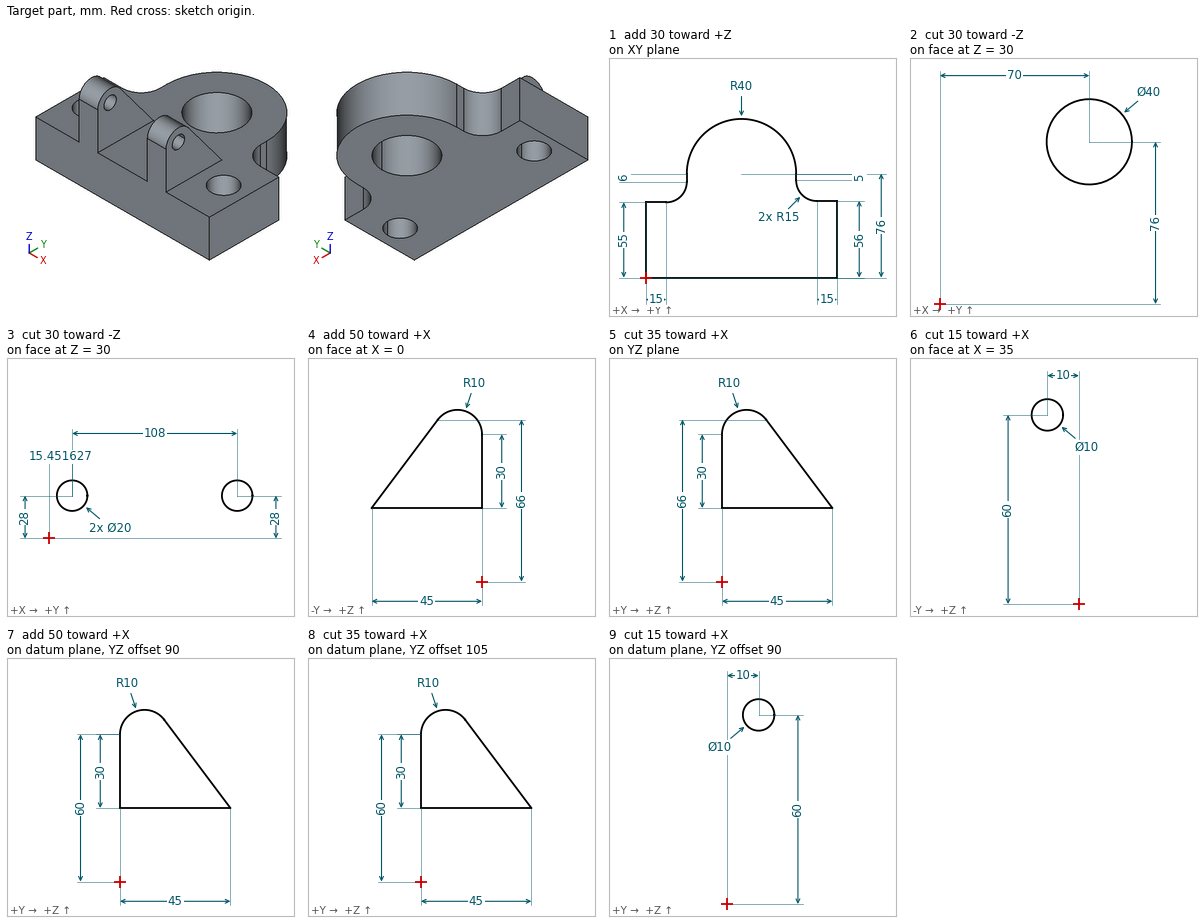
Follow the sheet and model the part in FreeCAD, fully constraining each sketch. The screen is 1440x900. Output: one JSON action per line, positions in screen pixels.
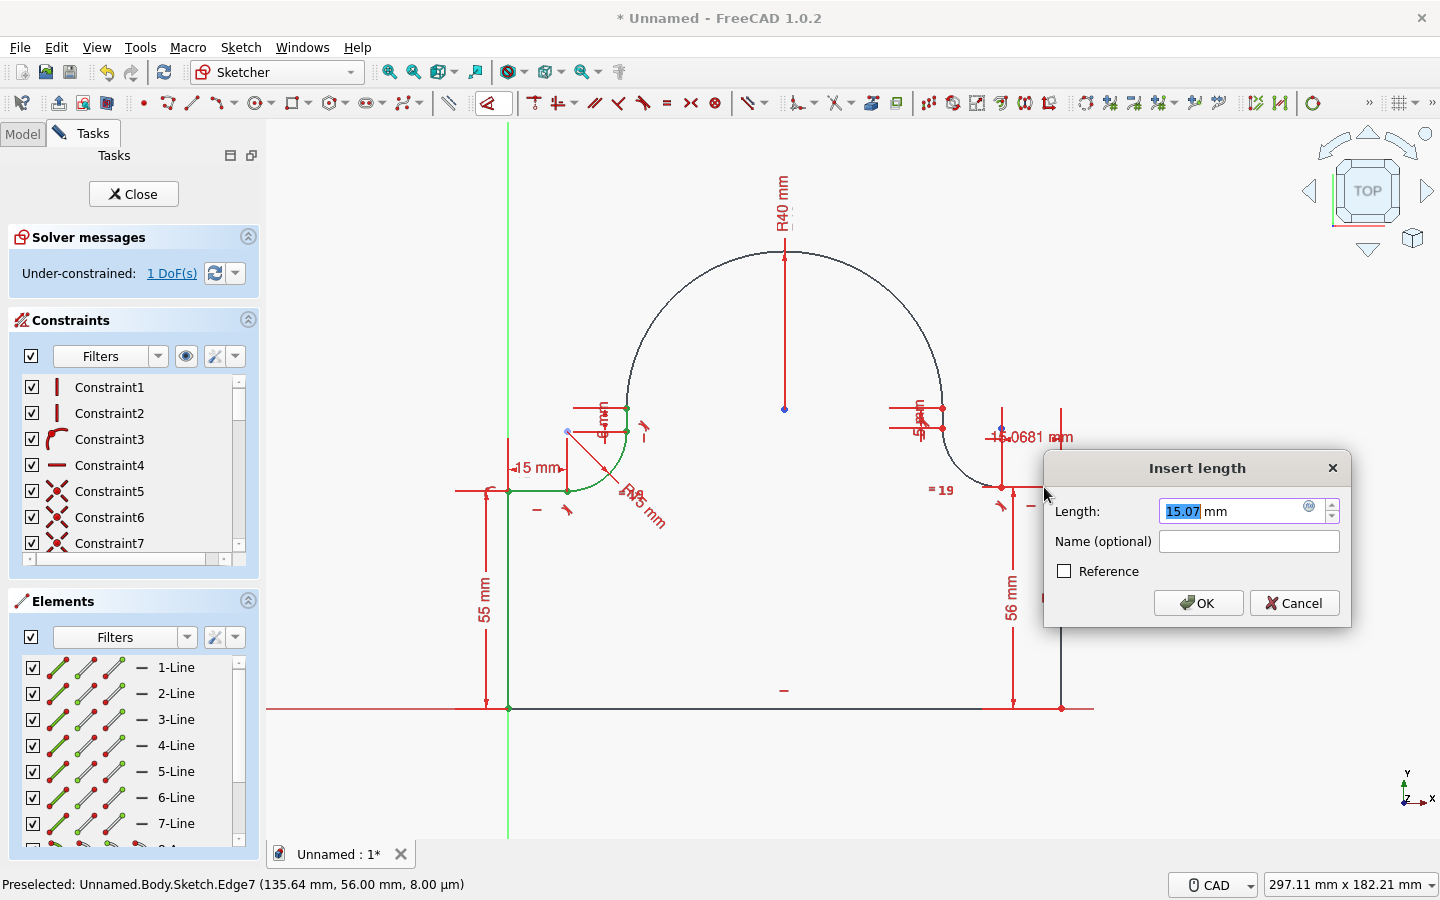
{"action": "type", "text": "15"}
{"action": "key", "text": "Return"}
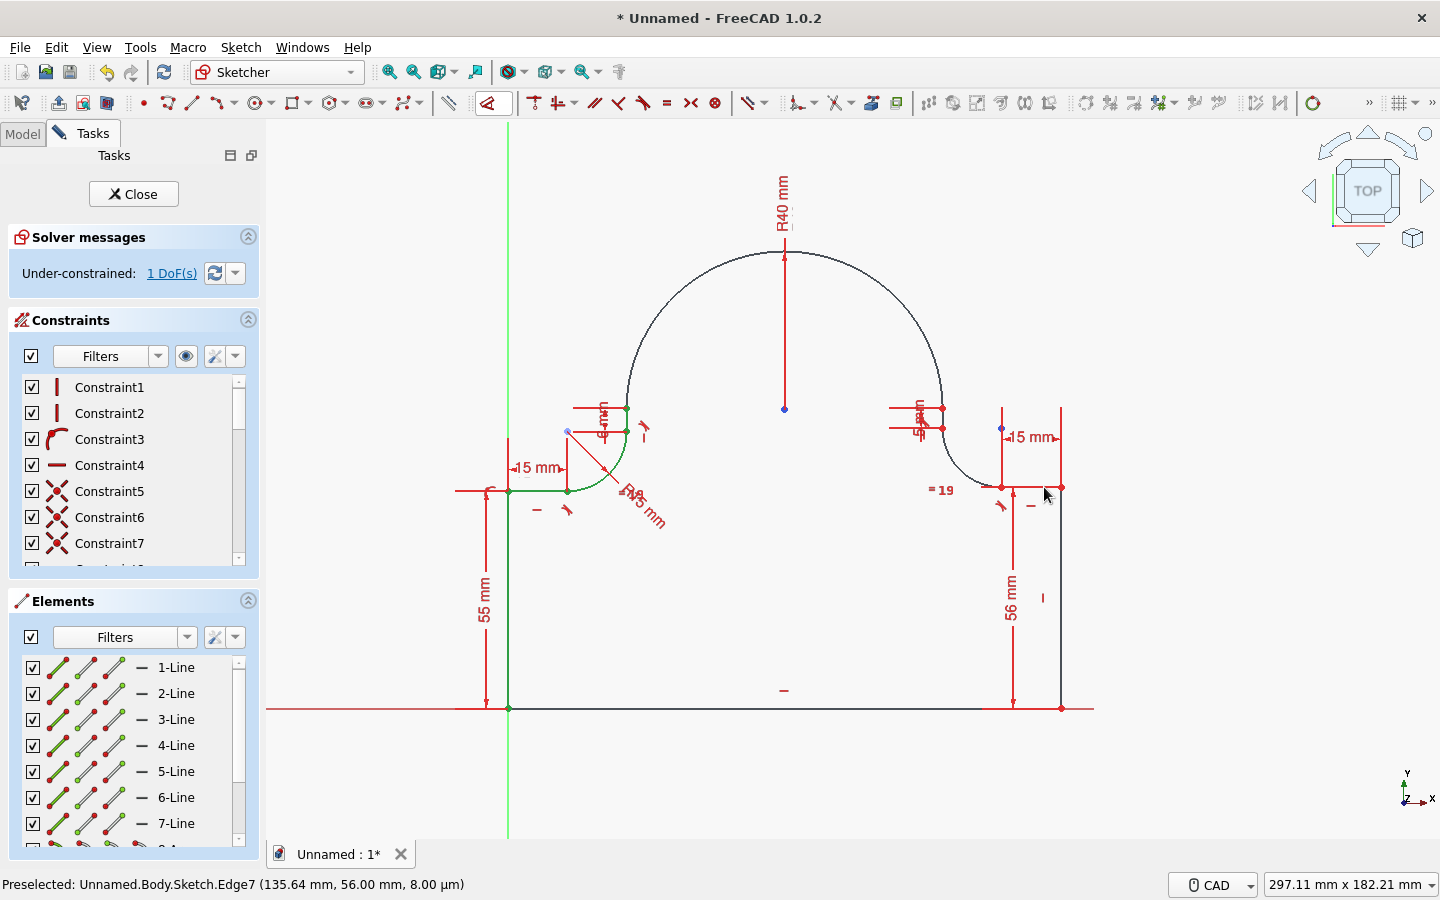
{"action": "left_click", "coordinate": [785, 410]}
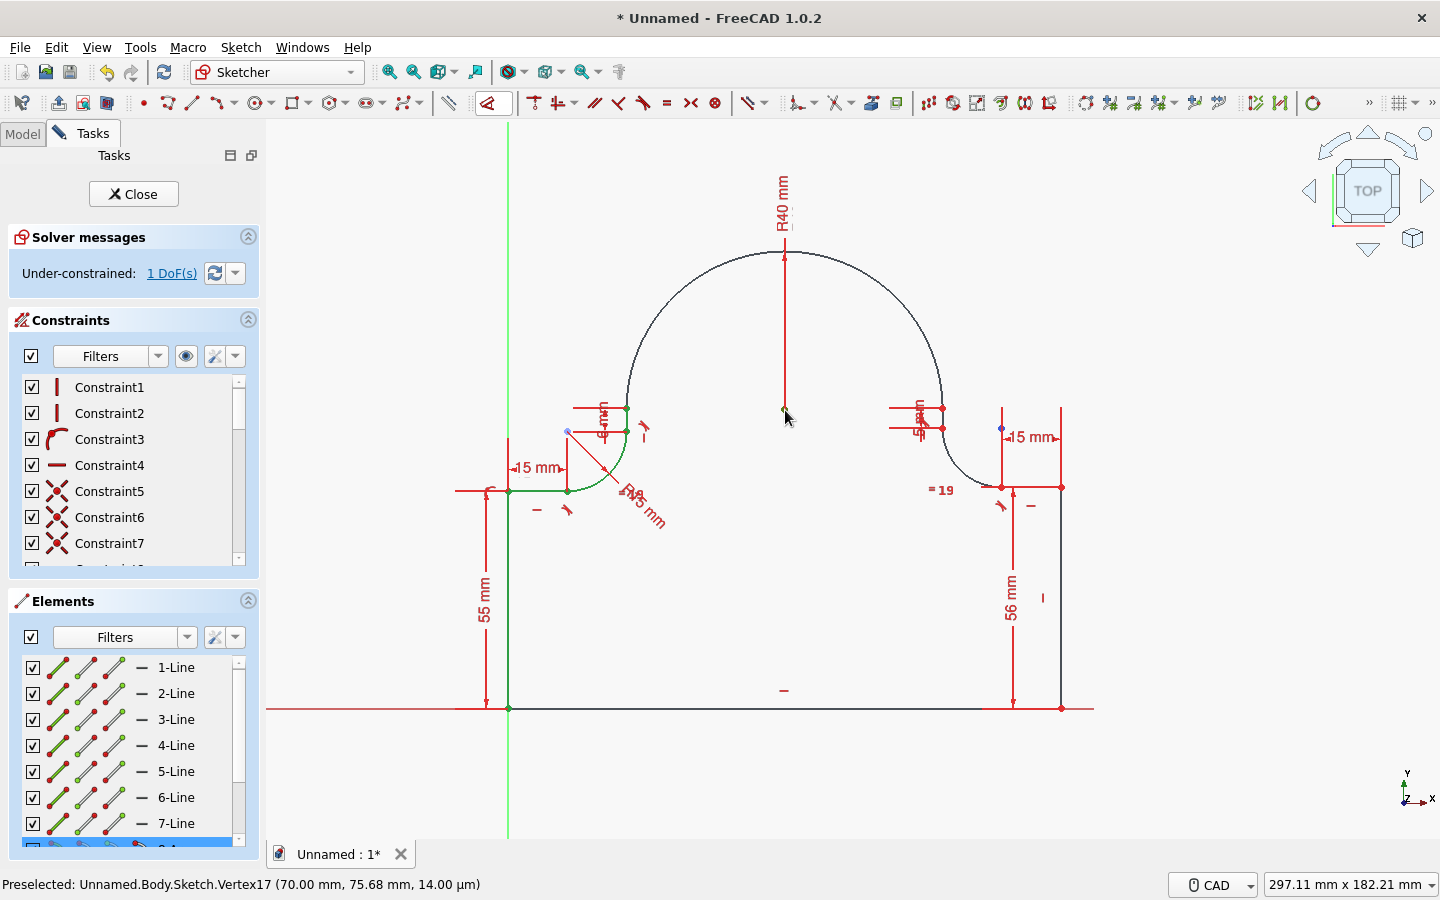
{"action": "key", "text": "i"}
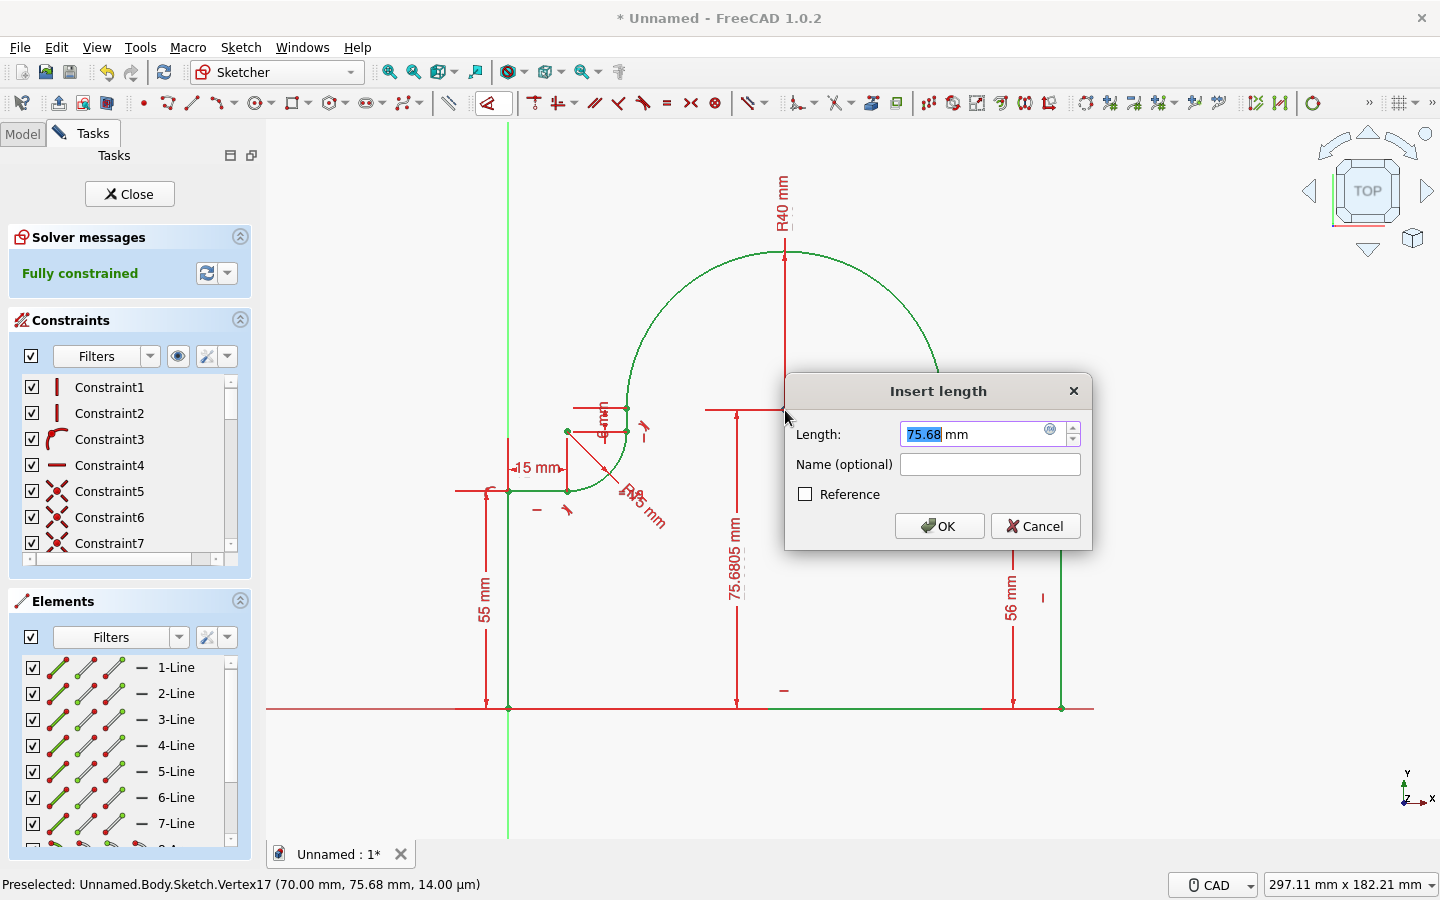
{"action": "type", "text": "76"}
{"action": "key", "text": "Return"}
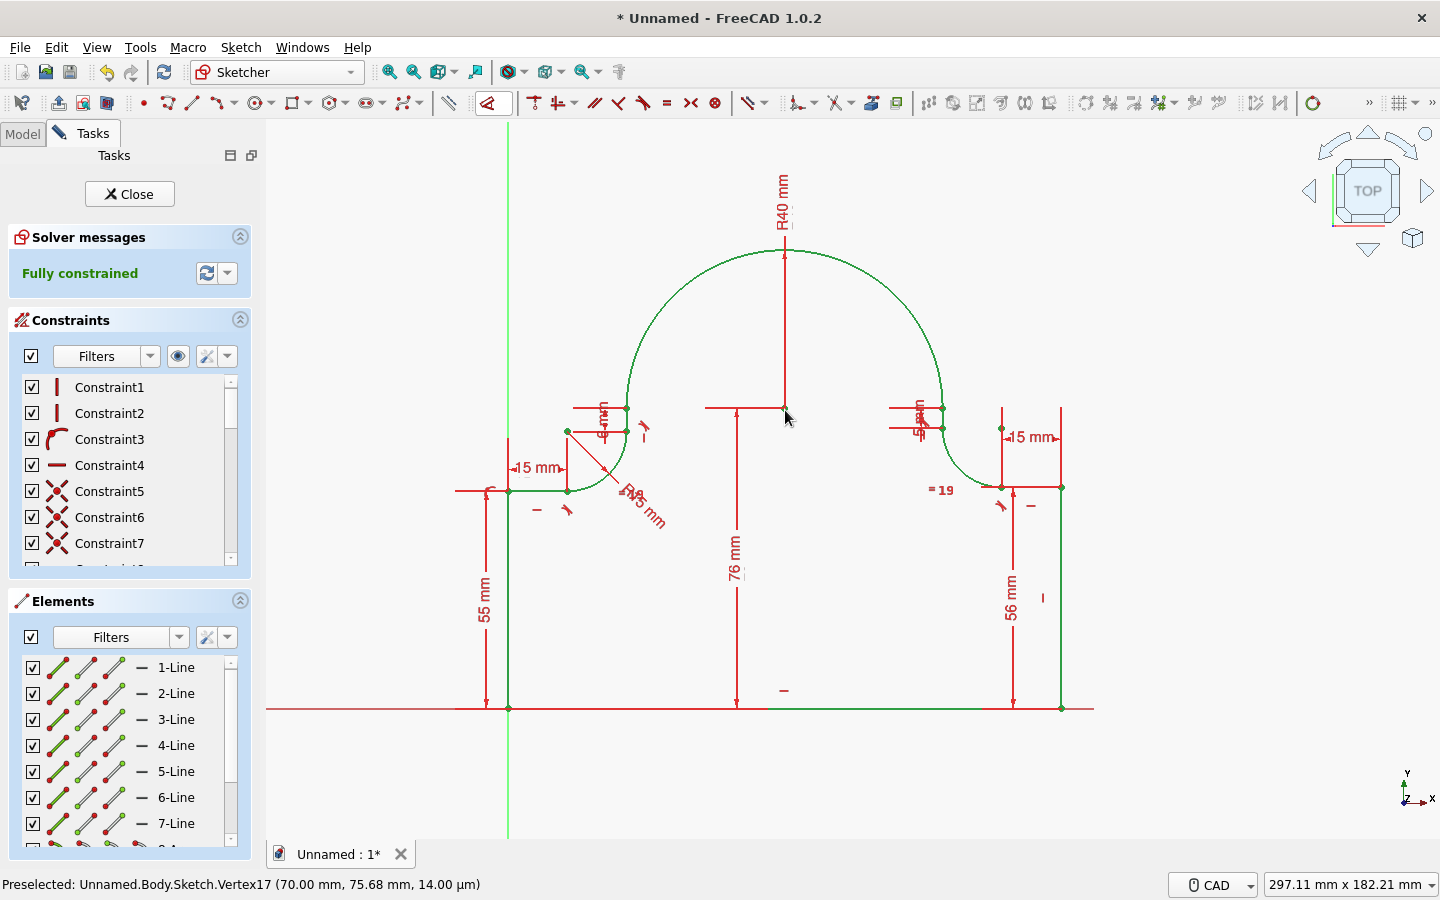
{"action": "left_click", "coordinate": [130, 194]}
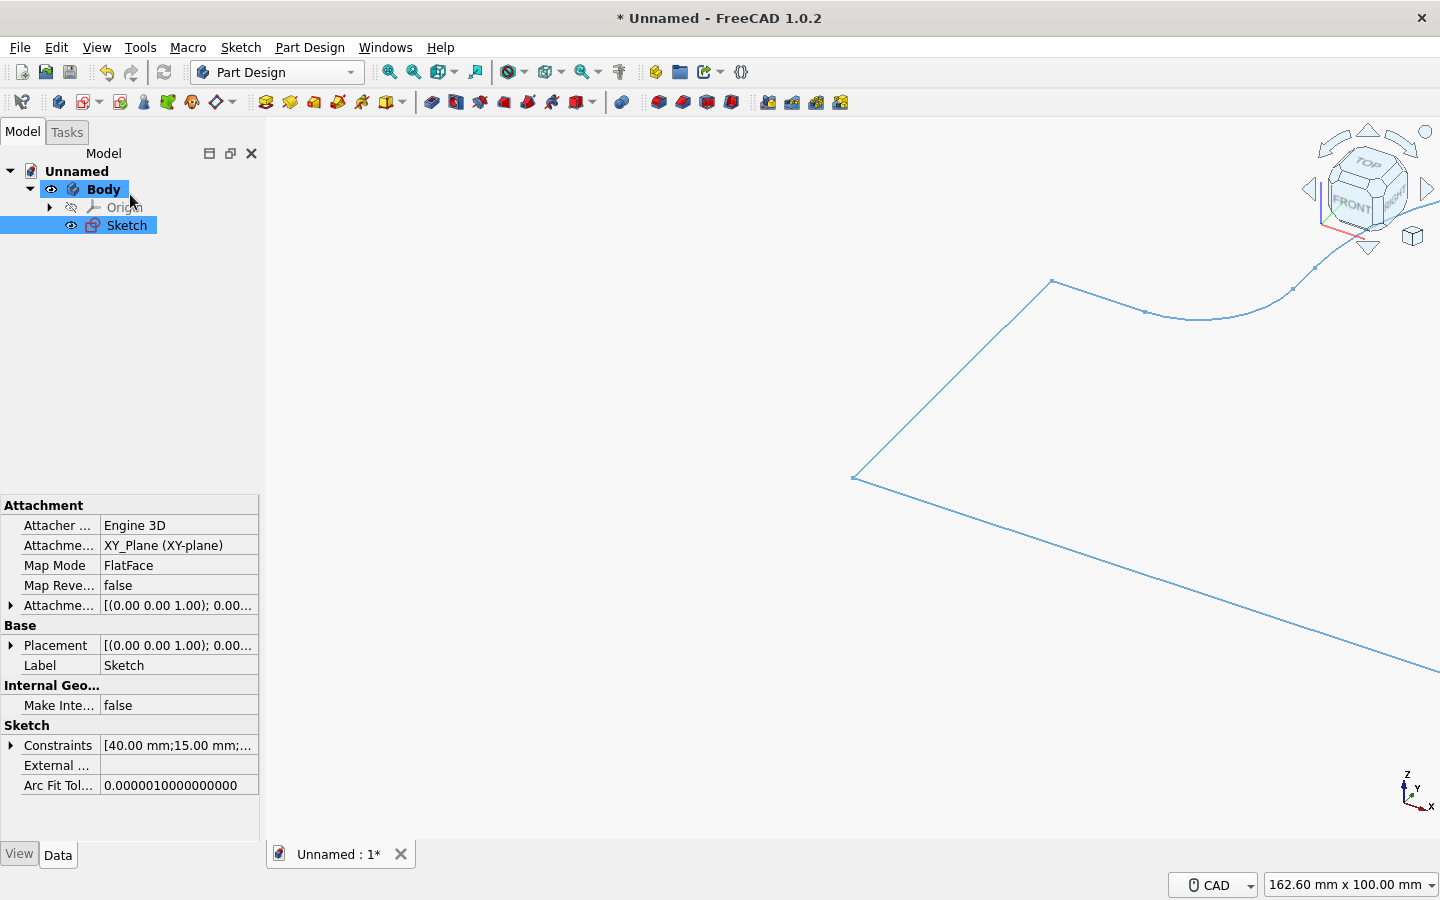
{"action": "left_click", "coordinate": [266, 102]}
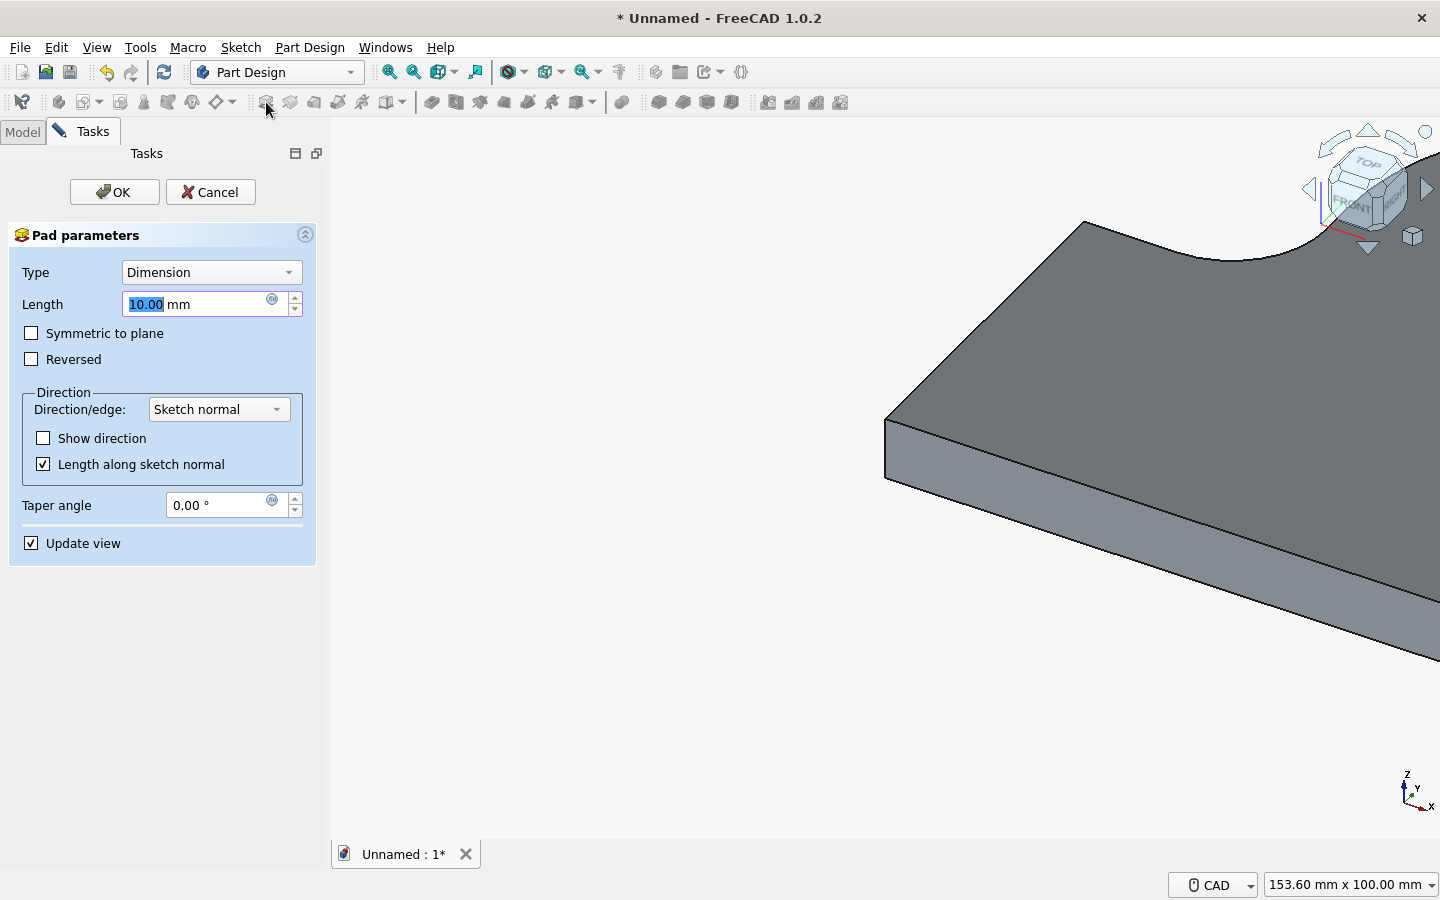
{"action": "type", "text": "30"}
{"action": "key", "text": "Tab"}